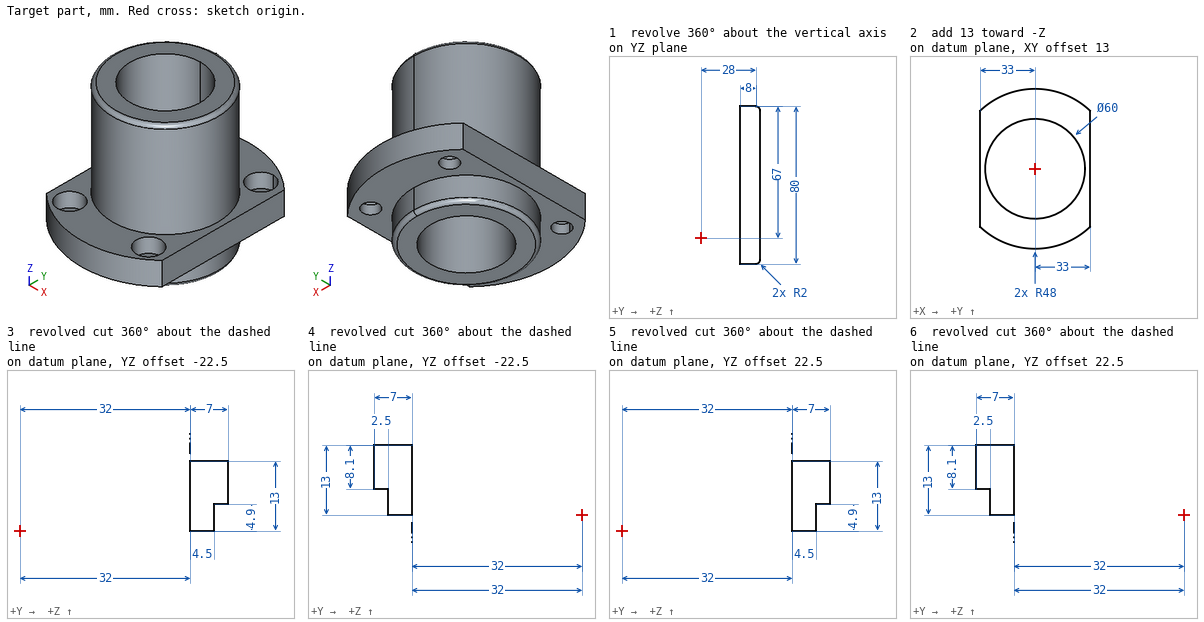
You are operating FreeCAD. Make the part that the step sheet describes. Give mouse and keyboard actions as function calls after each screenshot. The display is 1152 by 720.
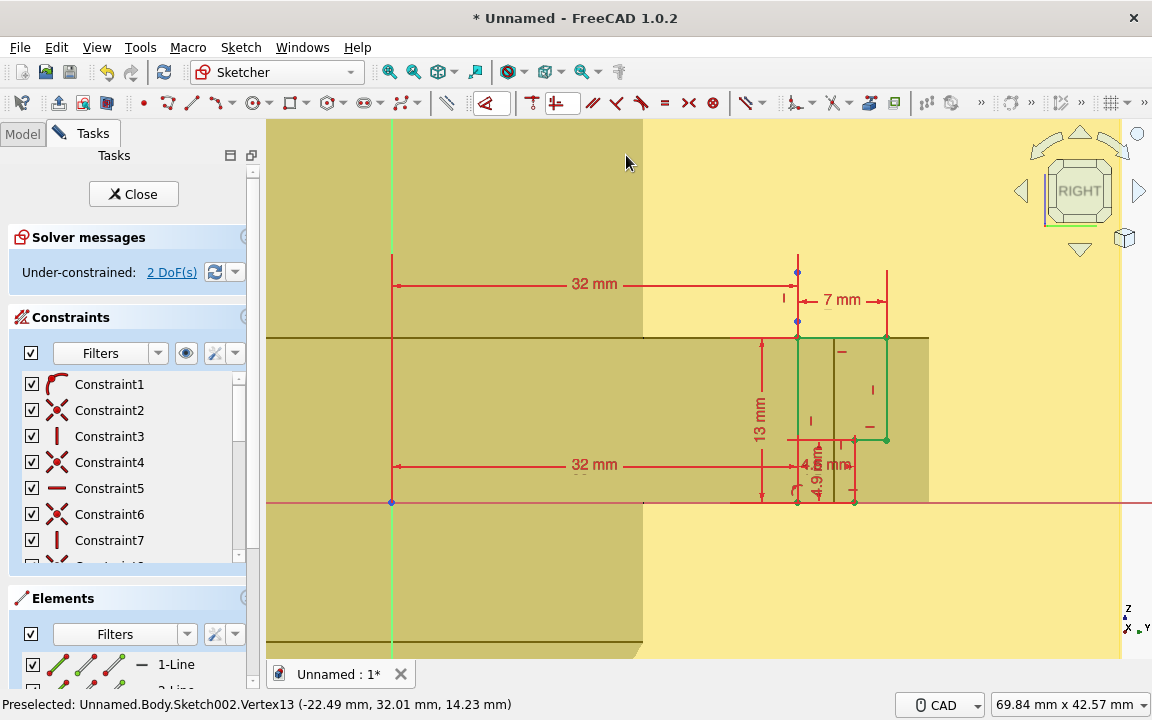
click(134, 194)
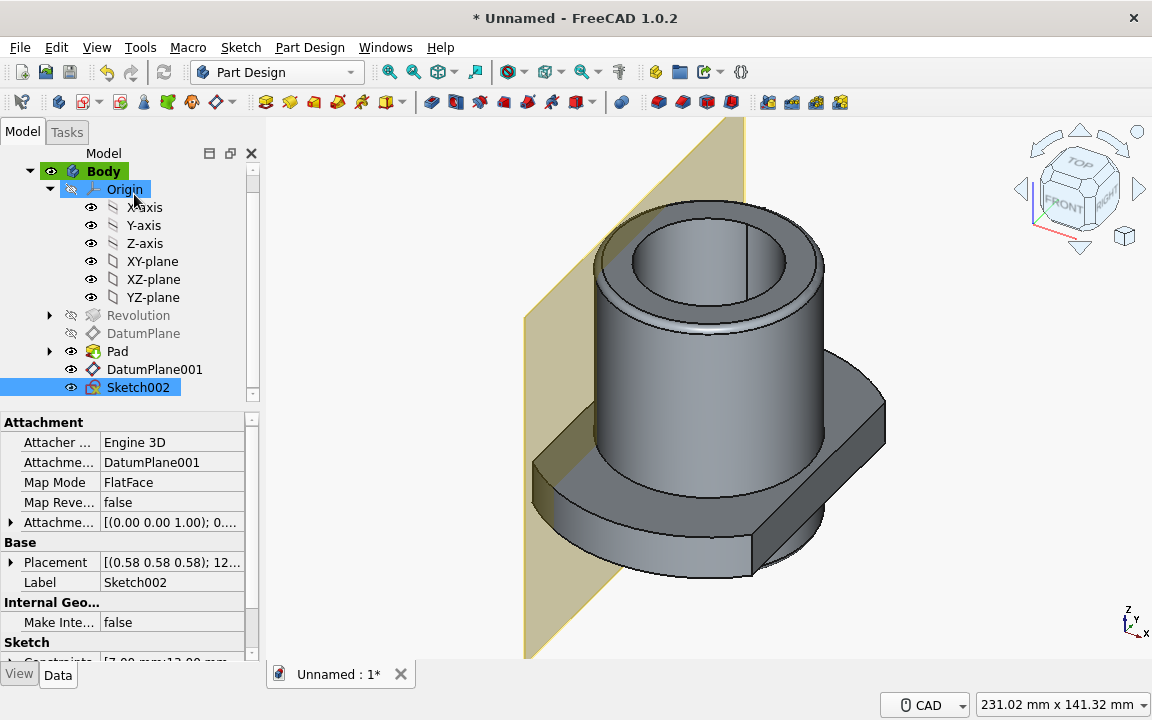
click(480, 102)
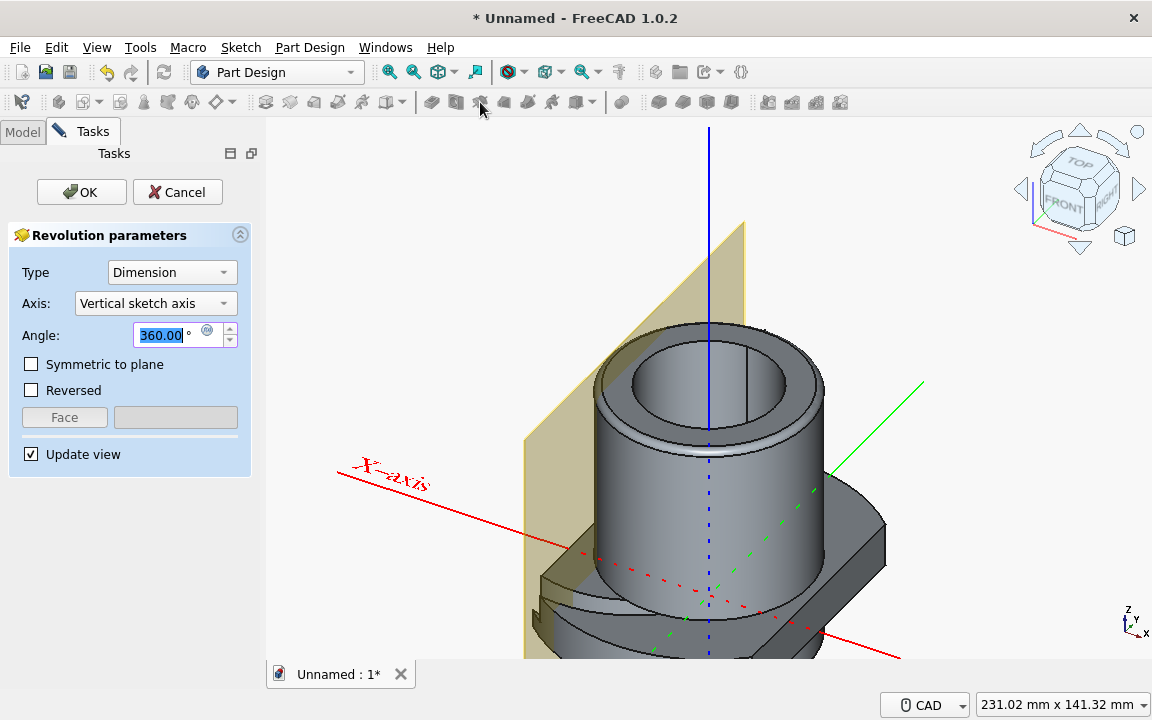
click(156, 304)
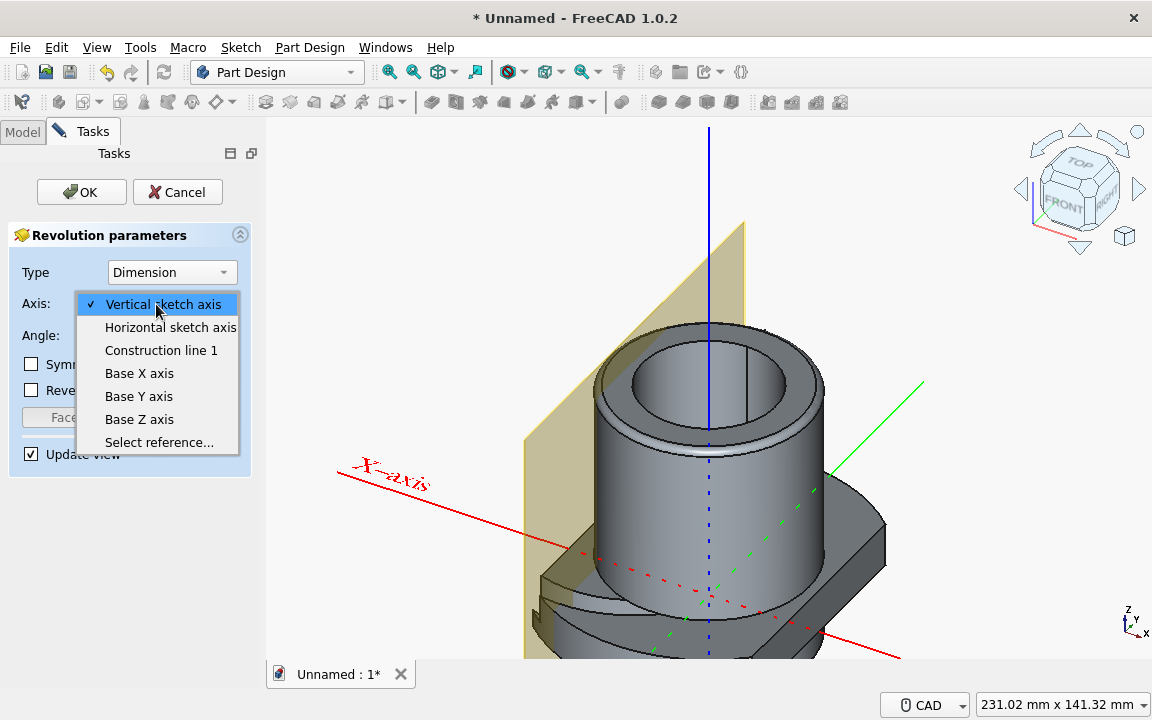
click(156, 350)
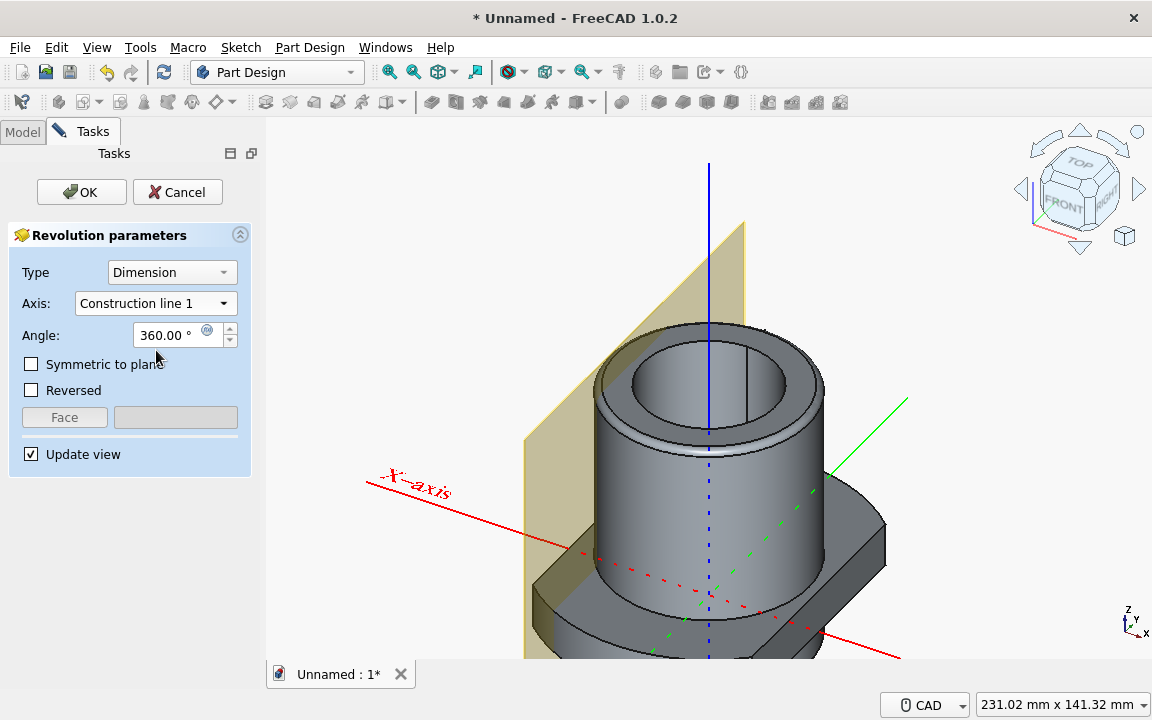
click(82, 192)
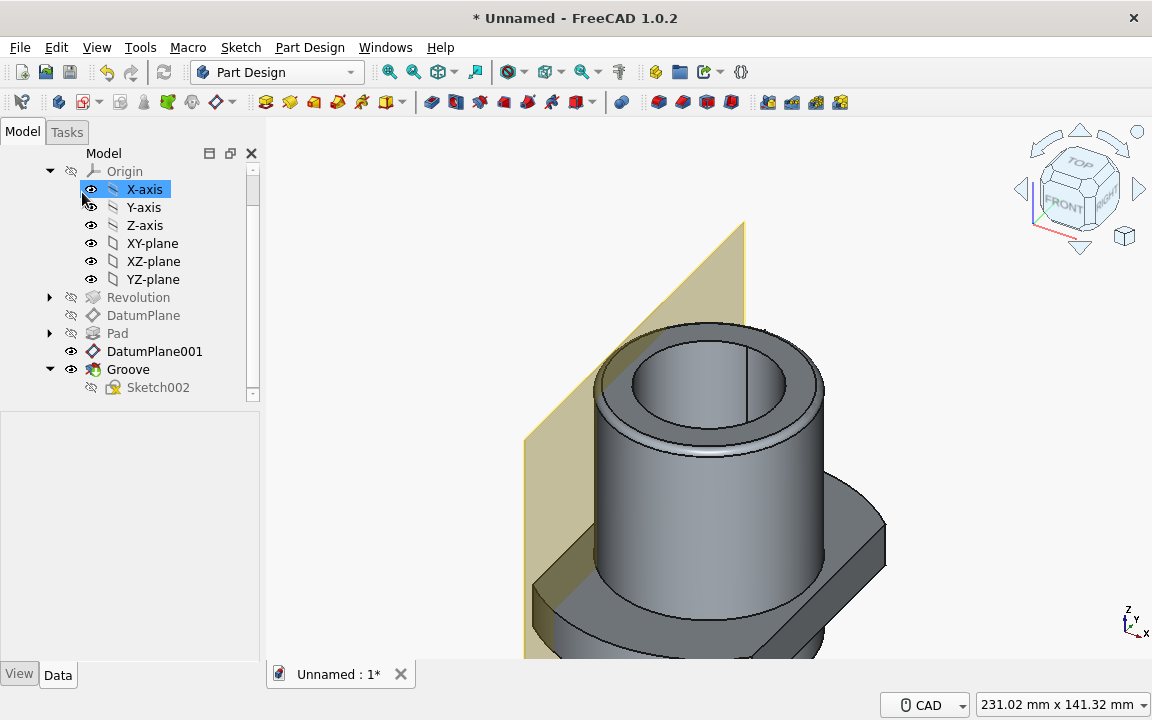
click(116, 351)
key(space)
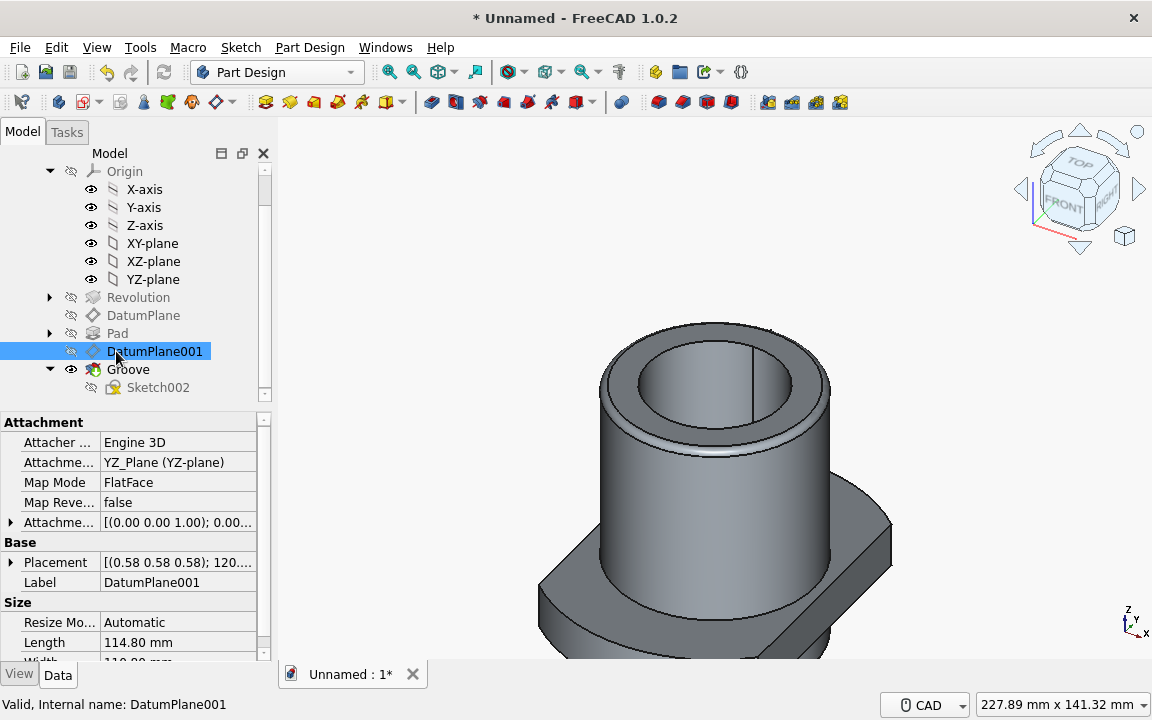
click(390, 72)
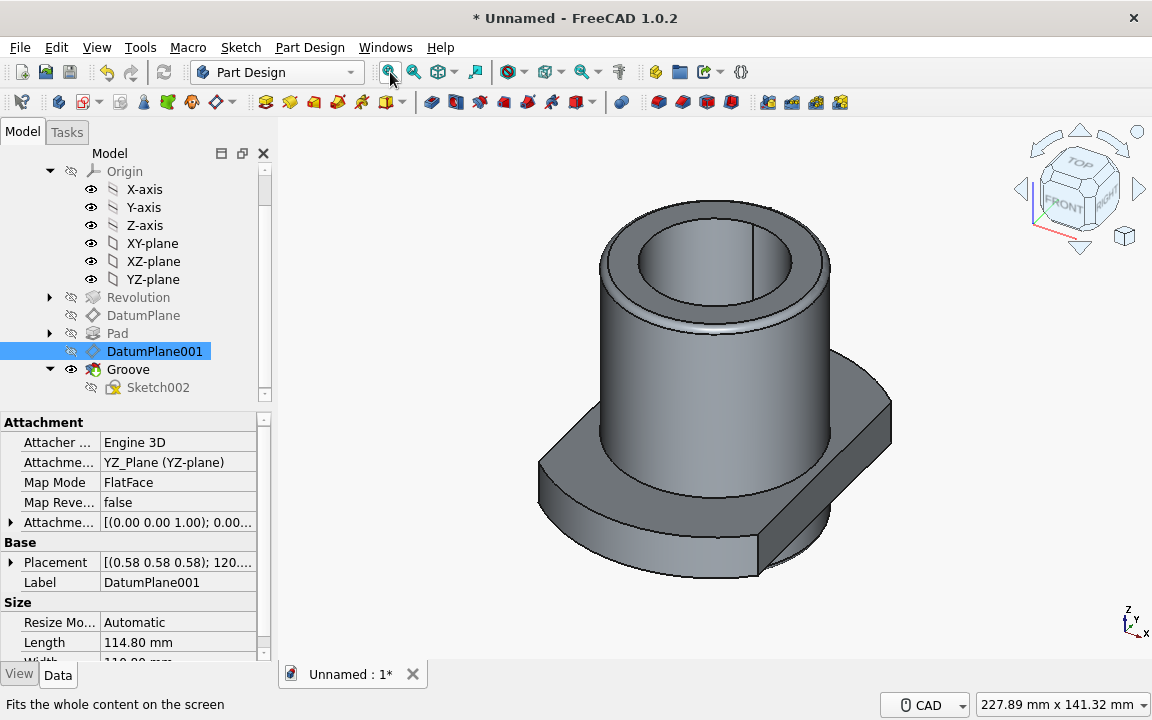
click(136, 279)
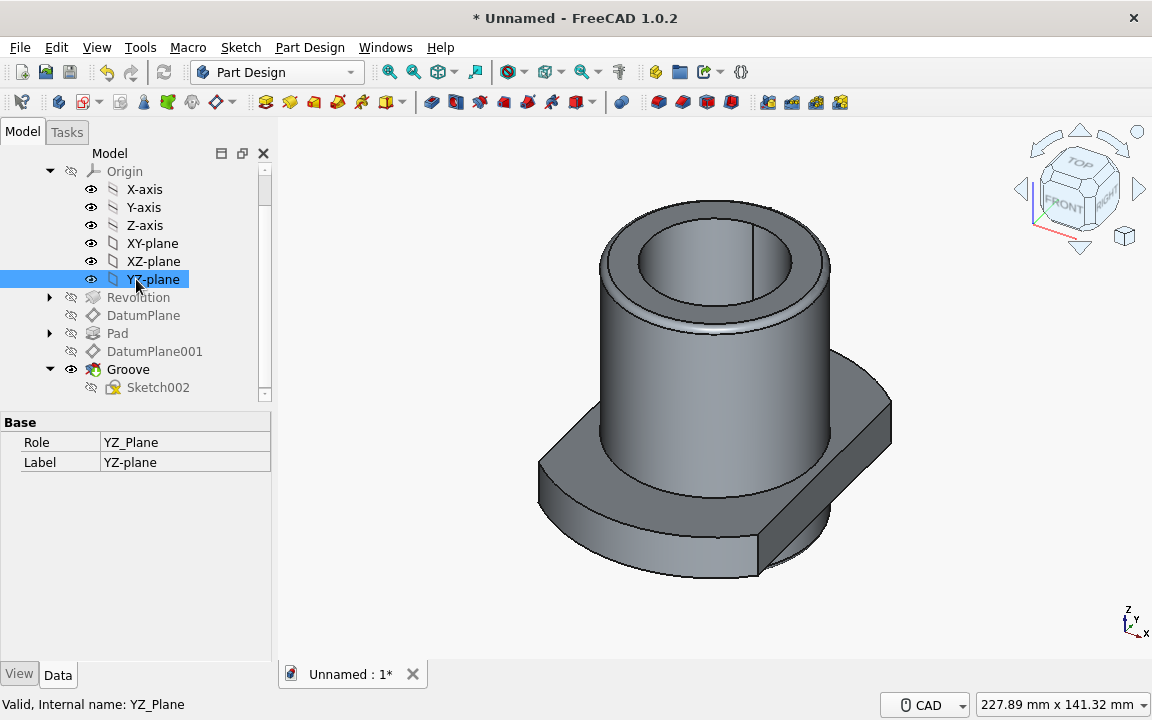
click(216, 102)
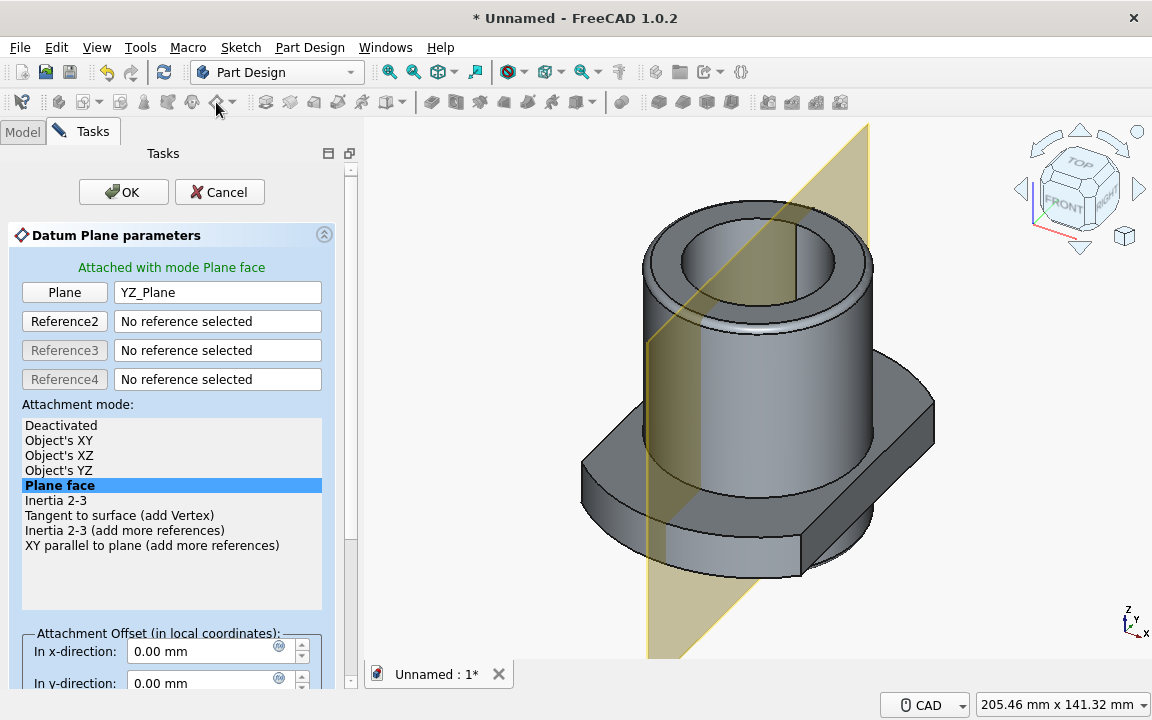
scroll(351, 426, down, 2)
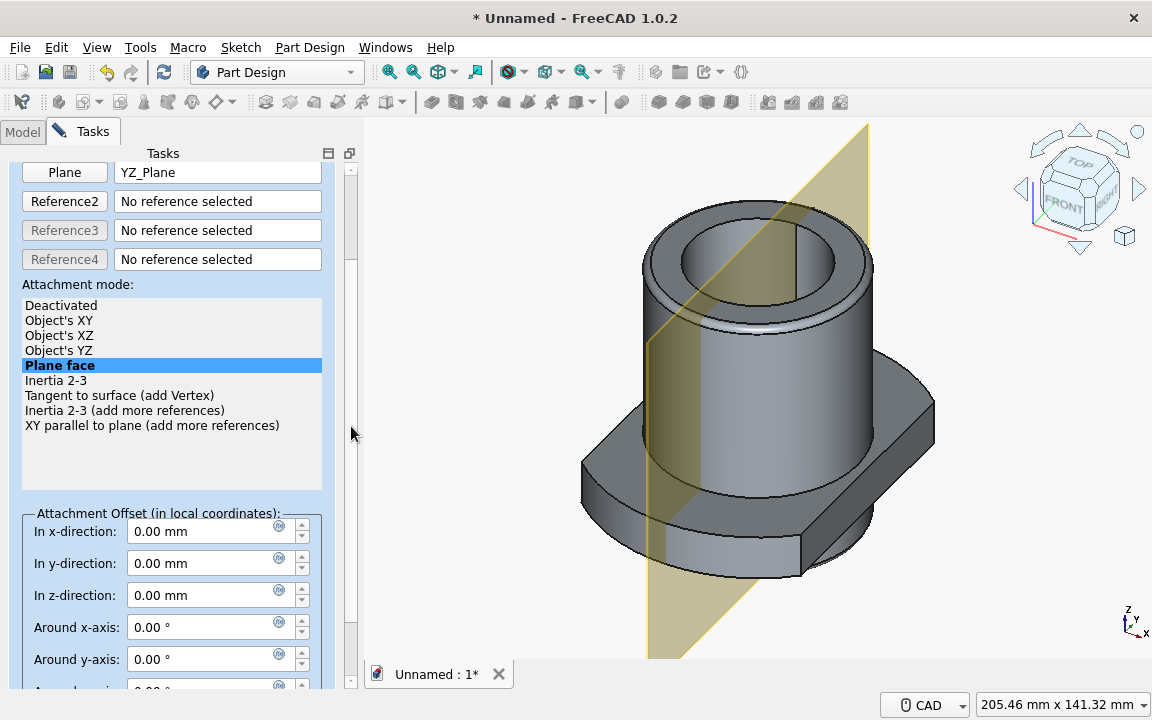
triple_click(210, 595)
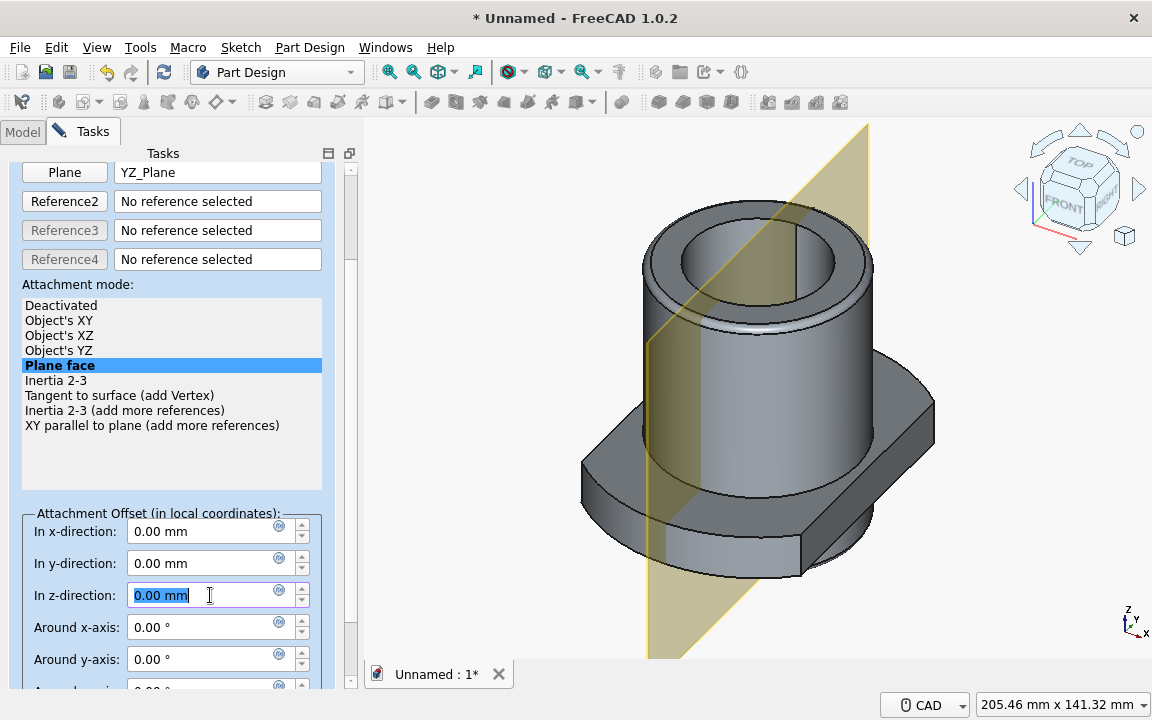
text(-22.5)
key(Tab)